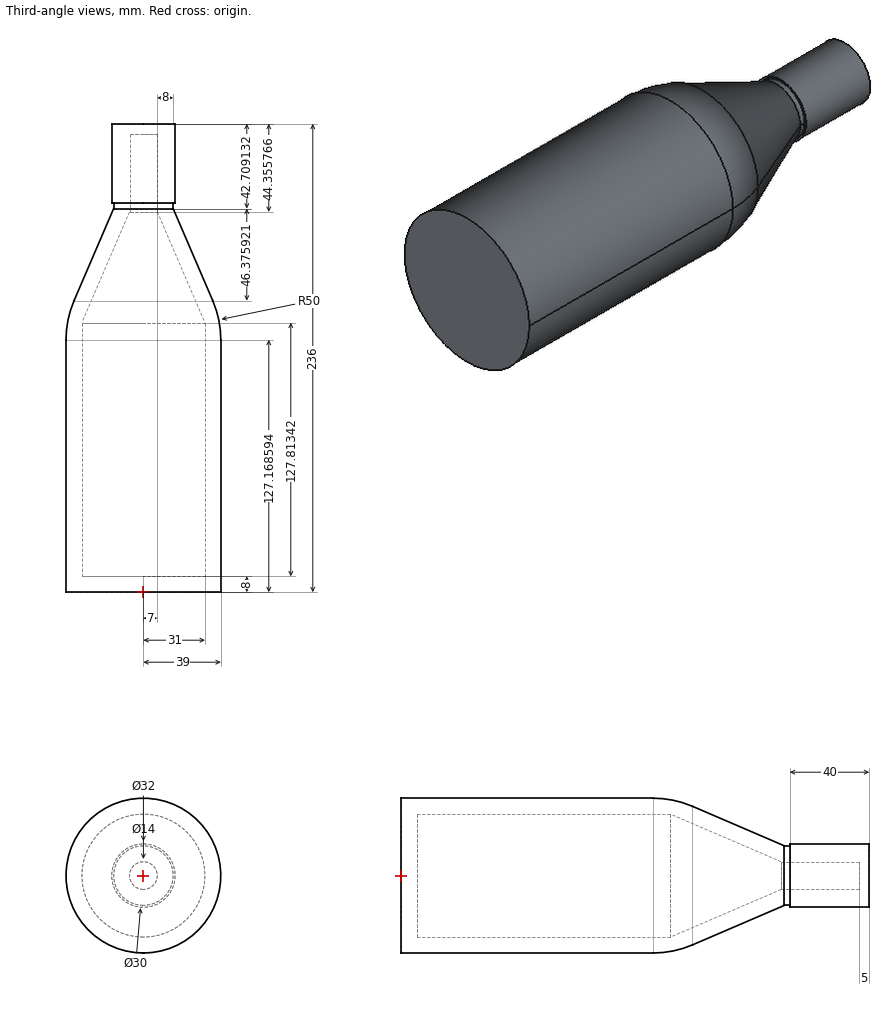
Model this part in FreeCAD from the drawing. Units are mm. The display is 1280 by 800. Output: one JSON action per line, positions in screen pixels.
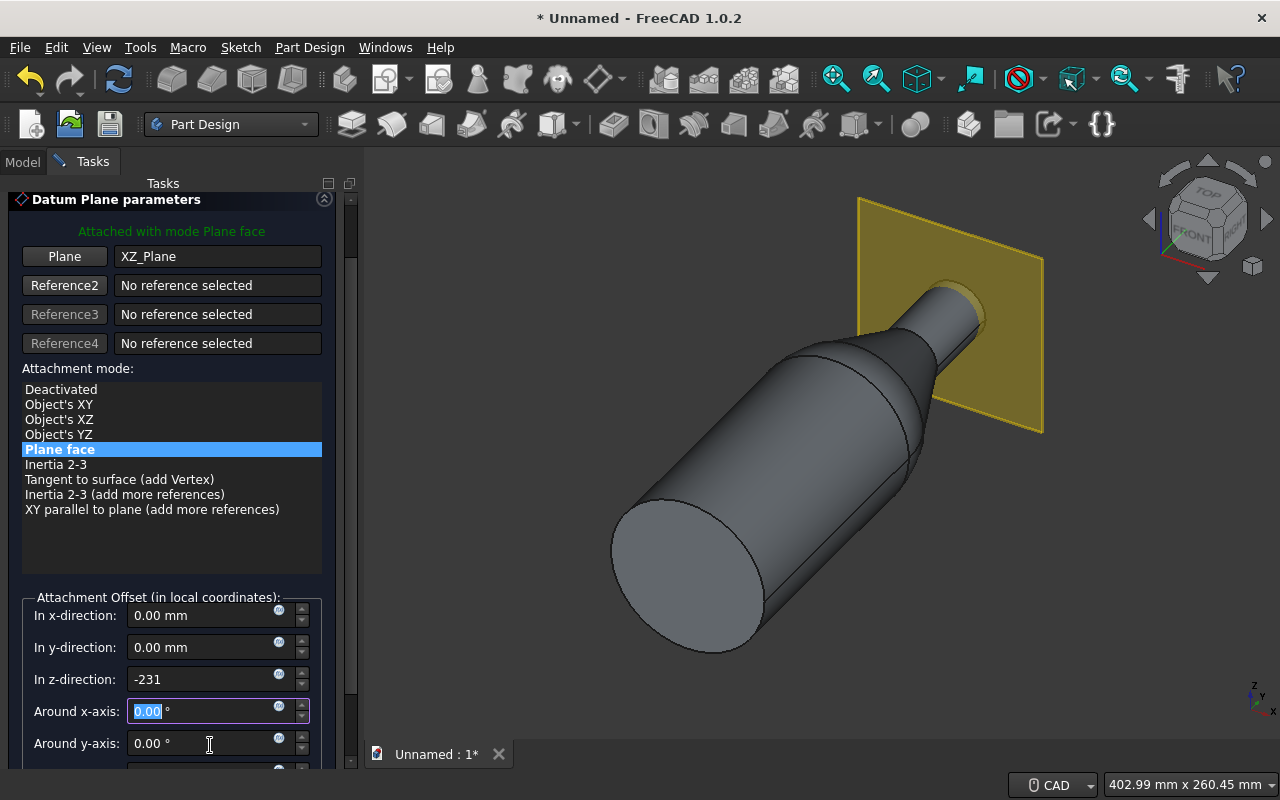
{"action": "scroll", "coordinate": [351, 480], "scroll_direction": "up", "scroll_amount": 2}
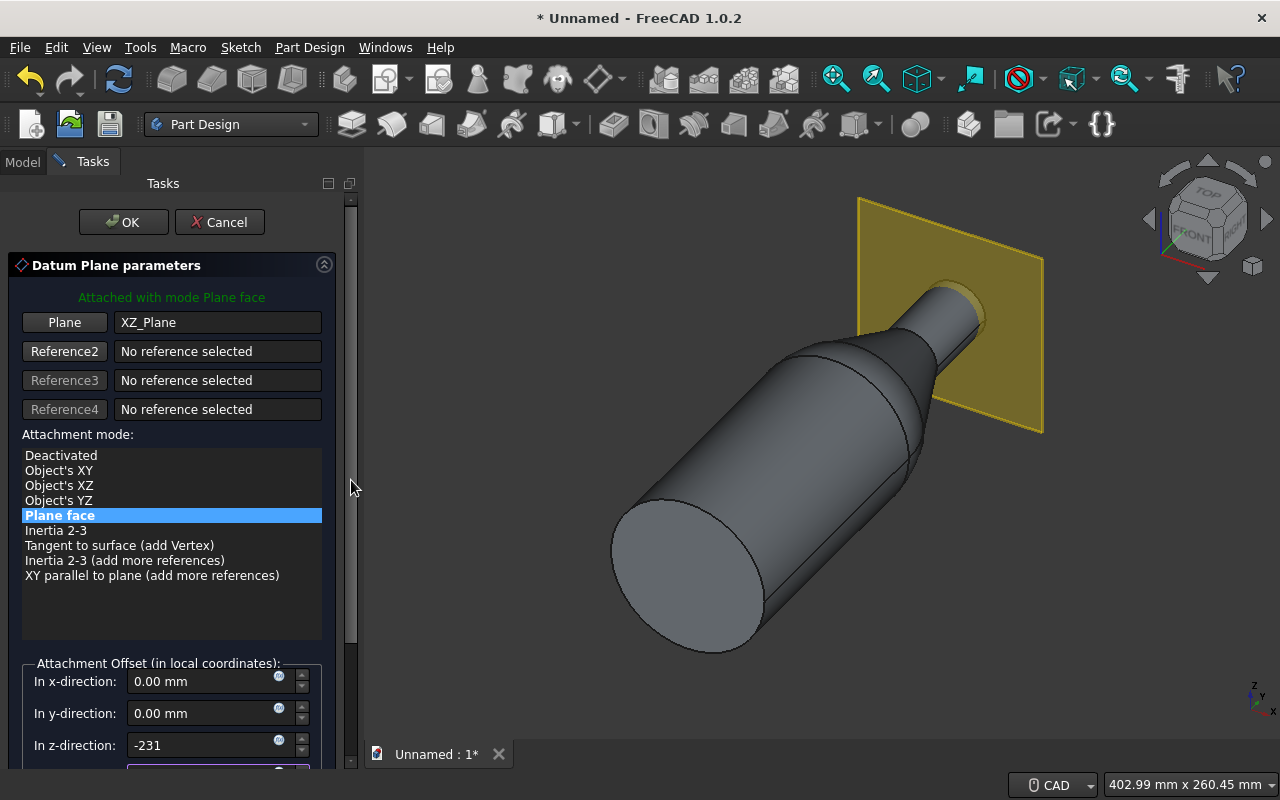
{"action": "left_click", "coordinate": [124, 222]}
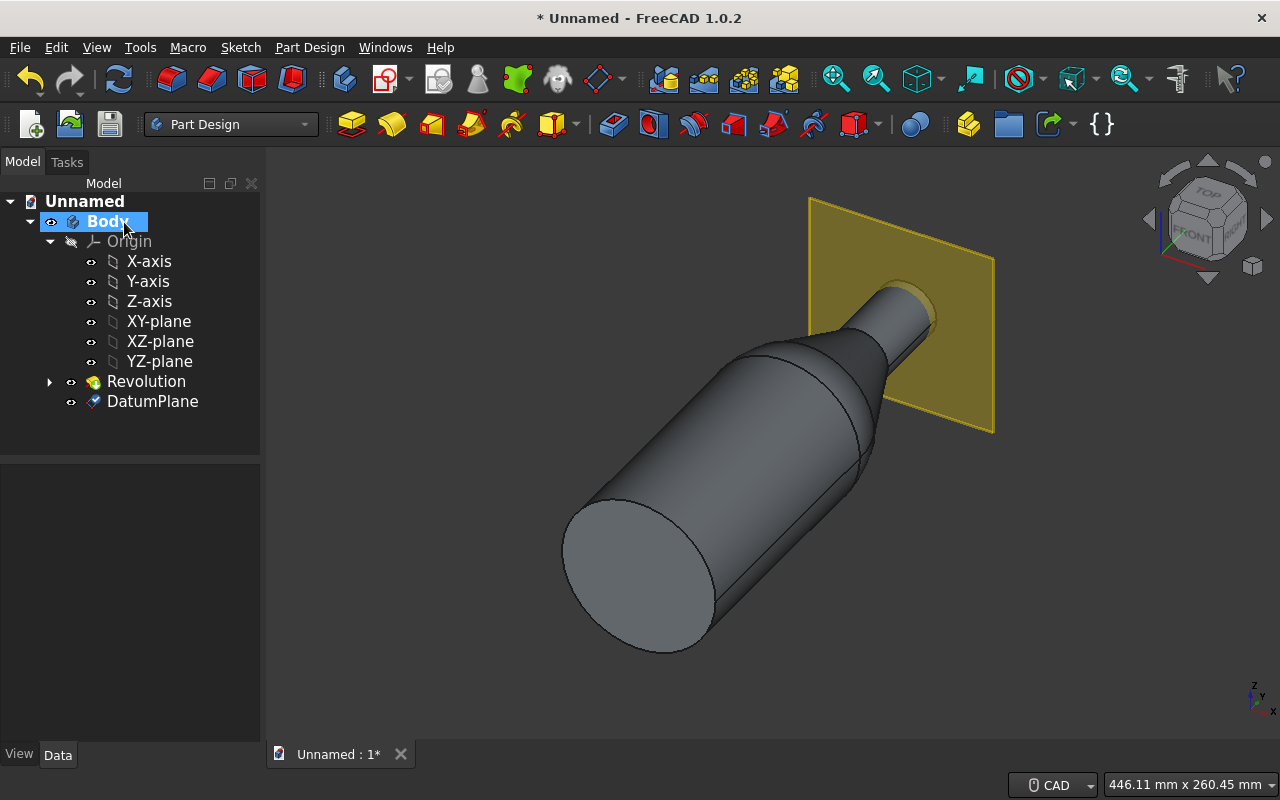
{"action": "left_click", "coordinate": [116, 402]}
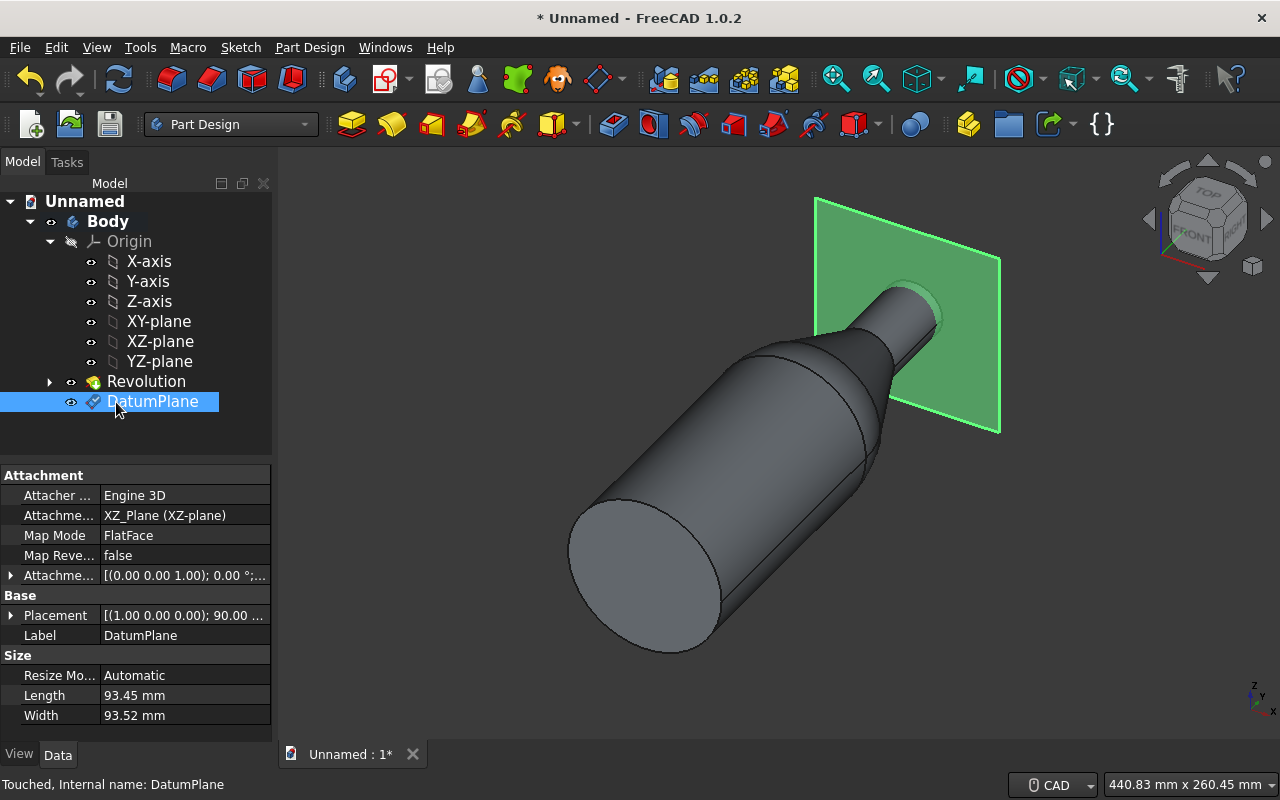
{"action": "left_click", "coordinate": [386, 80]}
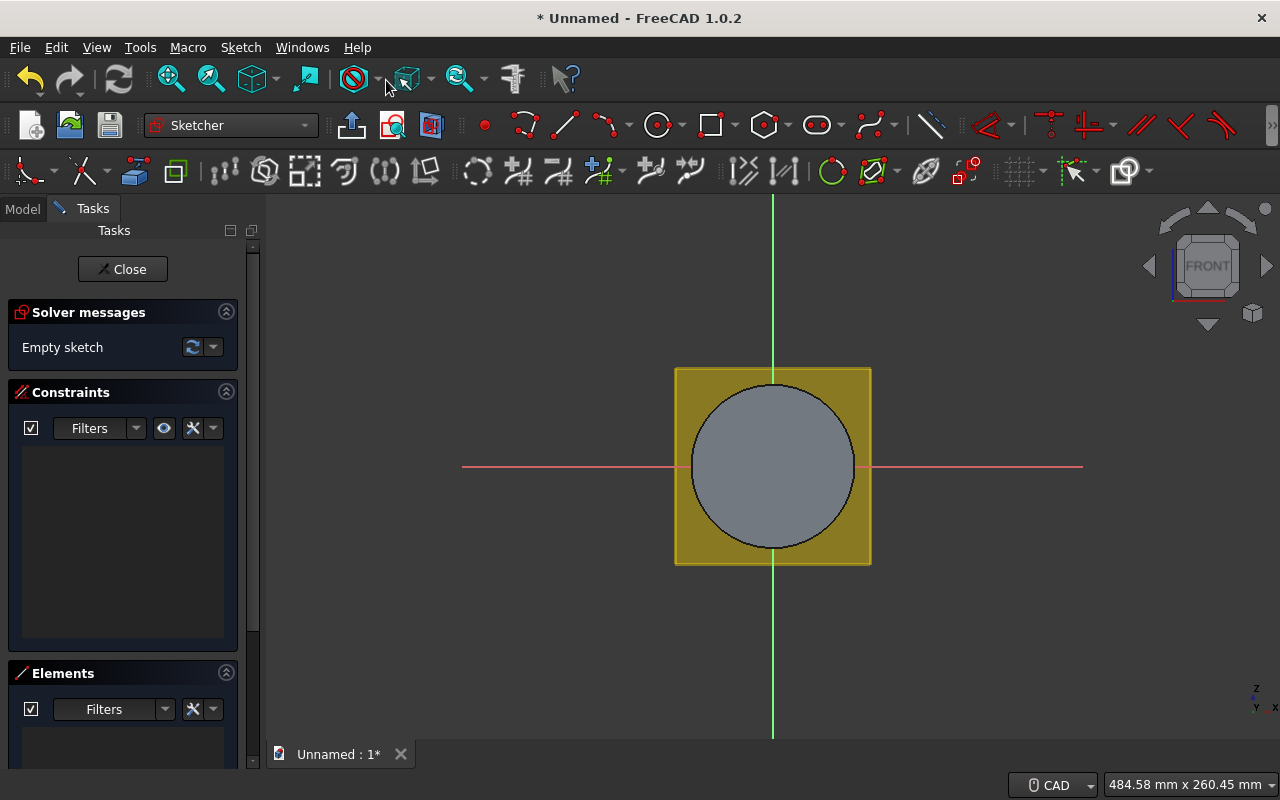
{"action": "key", "text": "q s"}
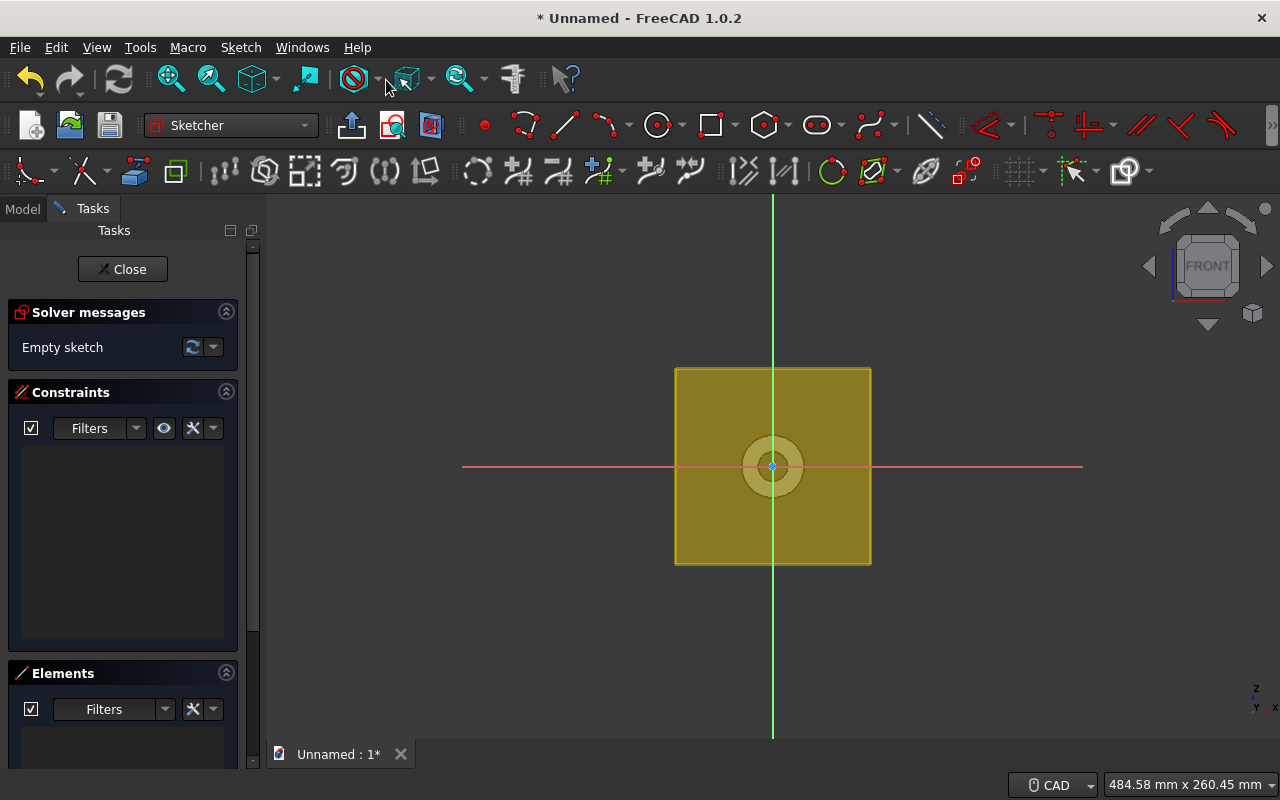
{"action": "scroll", "coordinate": [780, 467], "scroll_direction": "up", "scroll_amount": 12}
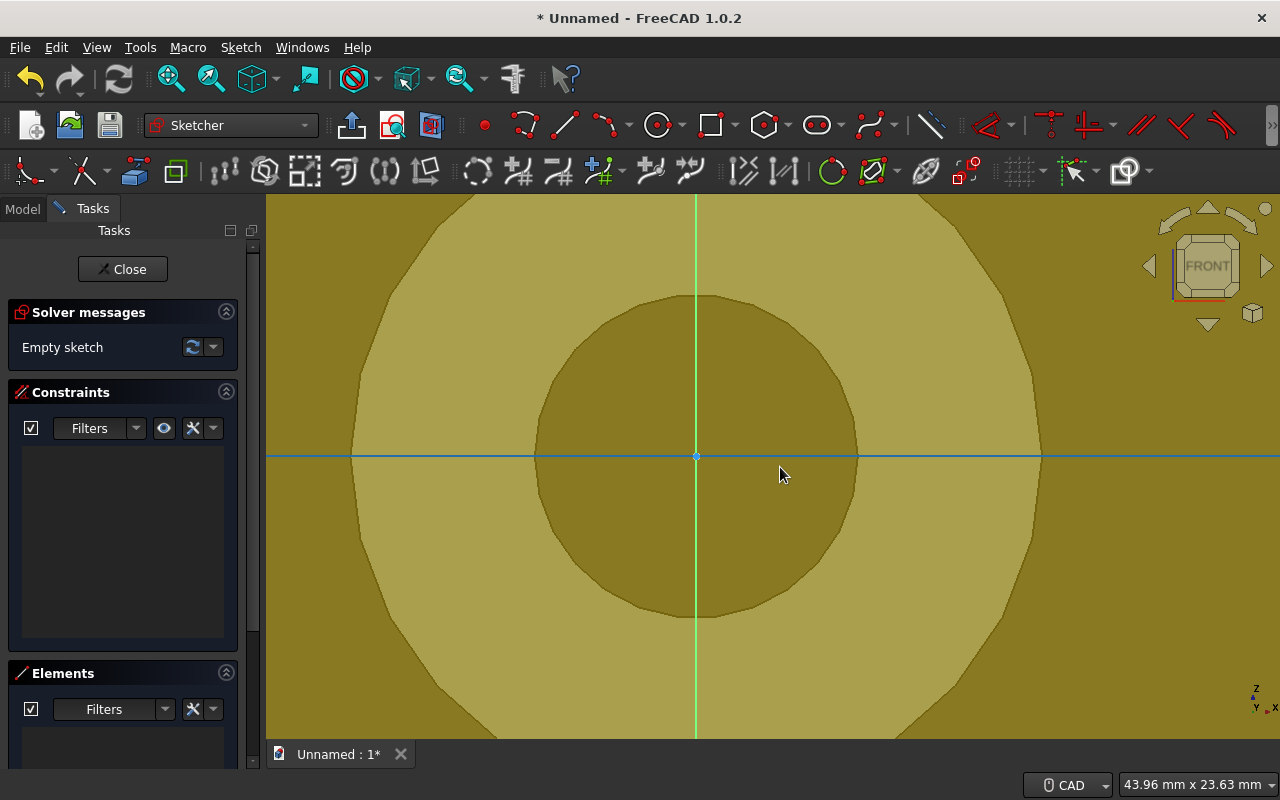
{"action": "key", "text": "g c"}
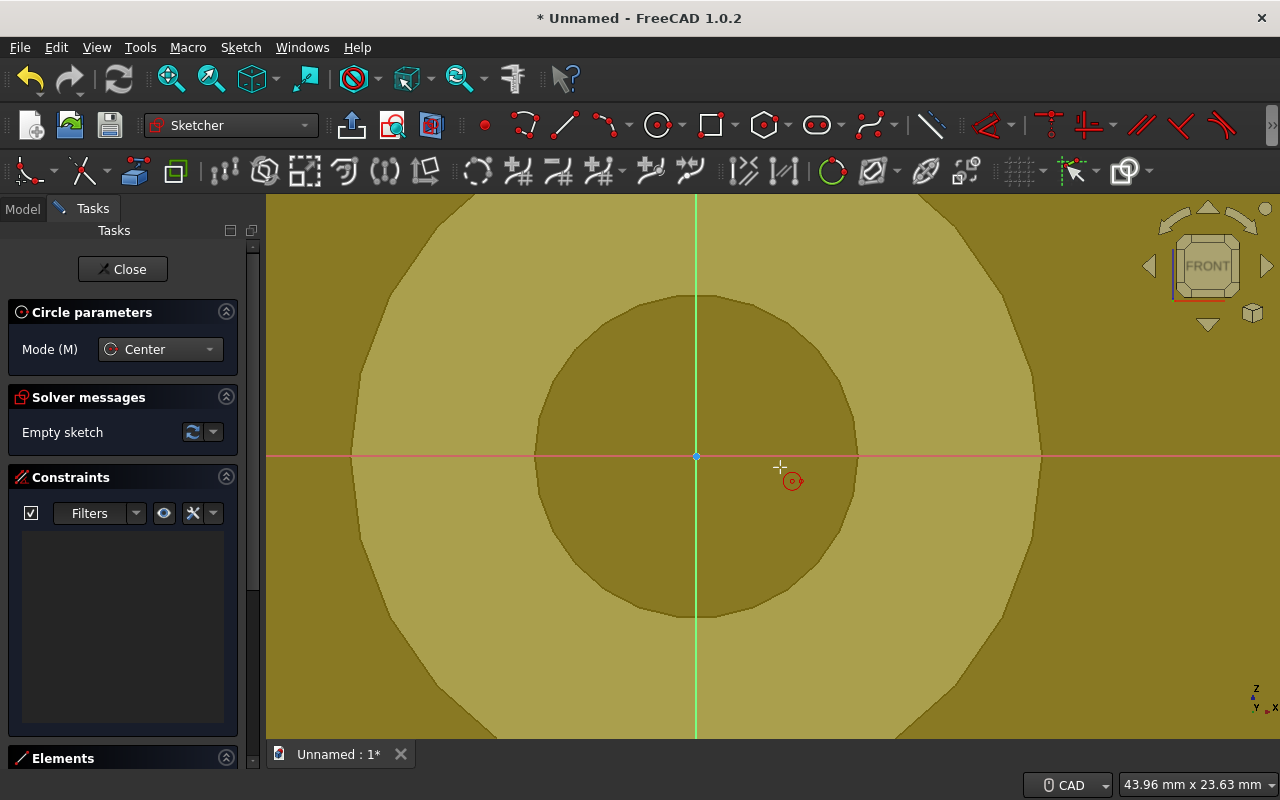
{"action": "left_click", "coordinate": [696, 456]}
{"action": "mouse_move", "coordinate": [810, 342]}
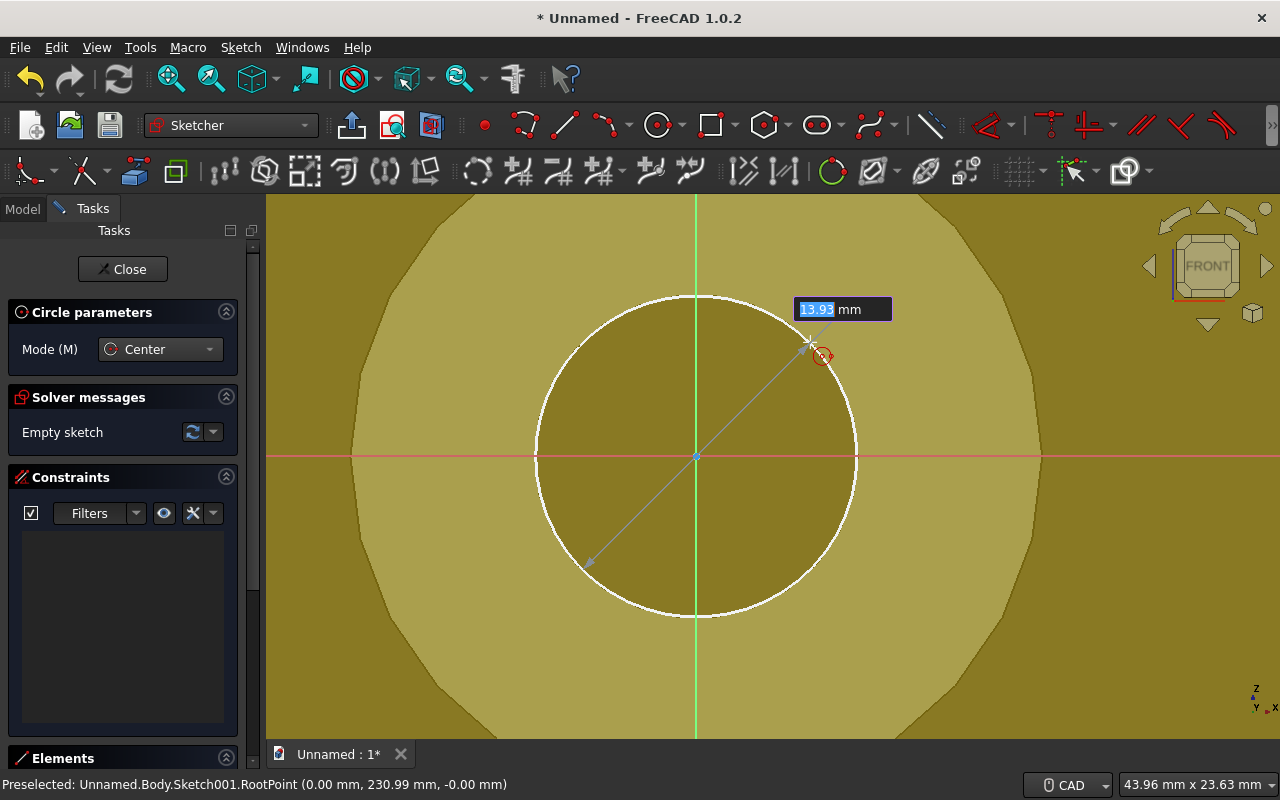
{"action": "type", "text": "14"}
{"action": "key", "text": "Return"}
{"action": "key", "text": "Escape"}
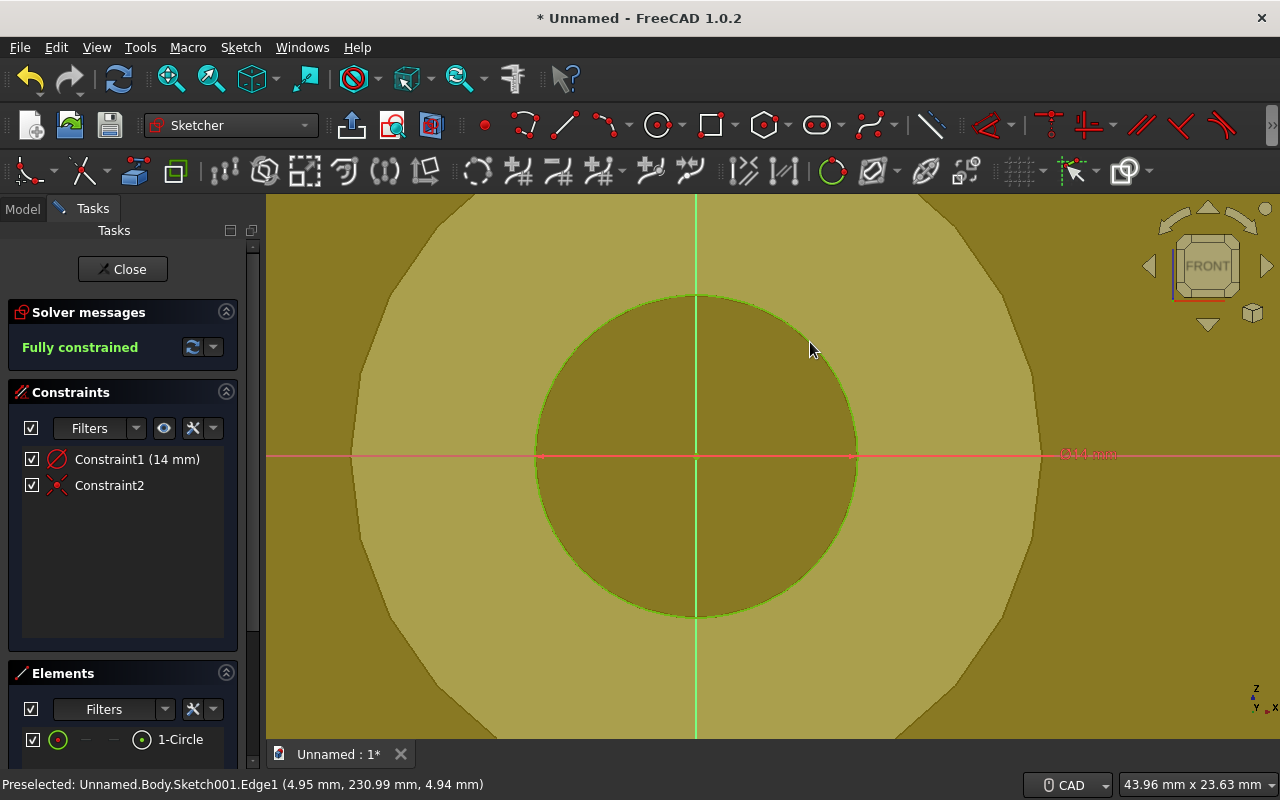
{"action": "left_click", "coordinate": [123, 269]}